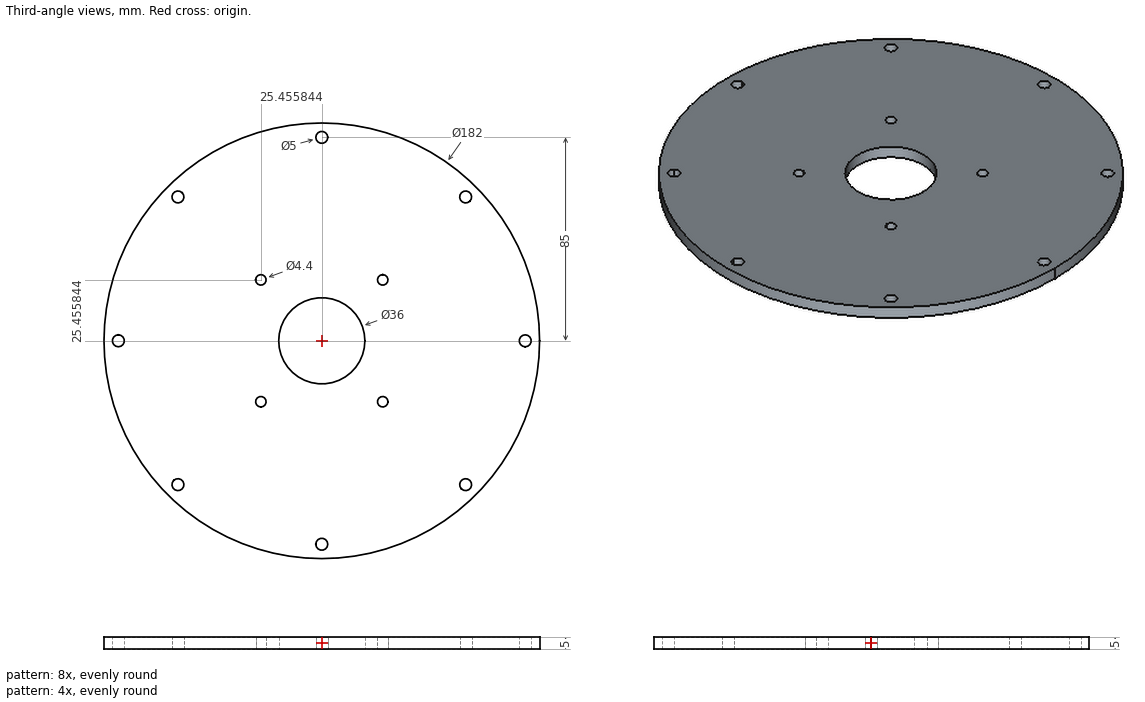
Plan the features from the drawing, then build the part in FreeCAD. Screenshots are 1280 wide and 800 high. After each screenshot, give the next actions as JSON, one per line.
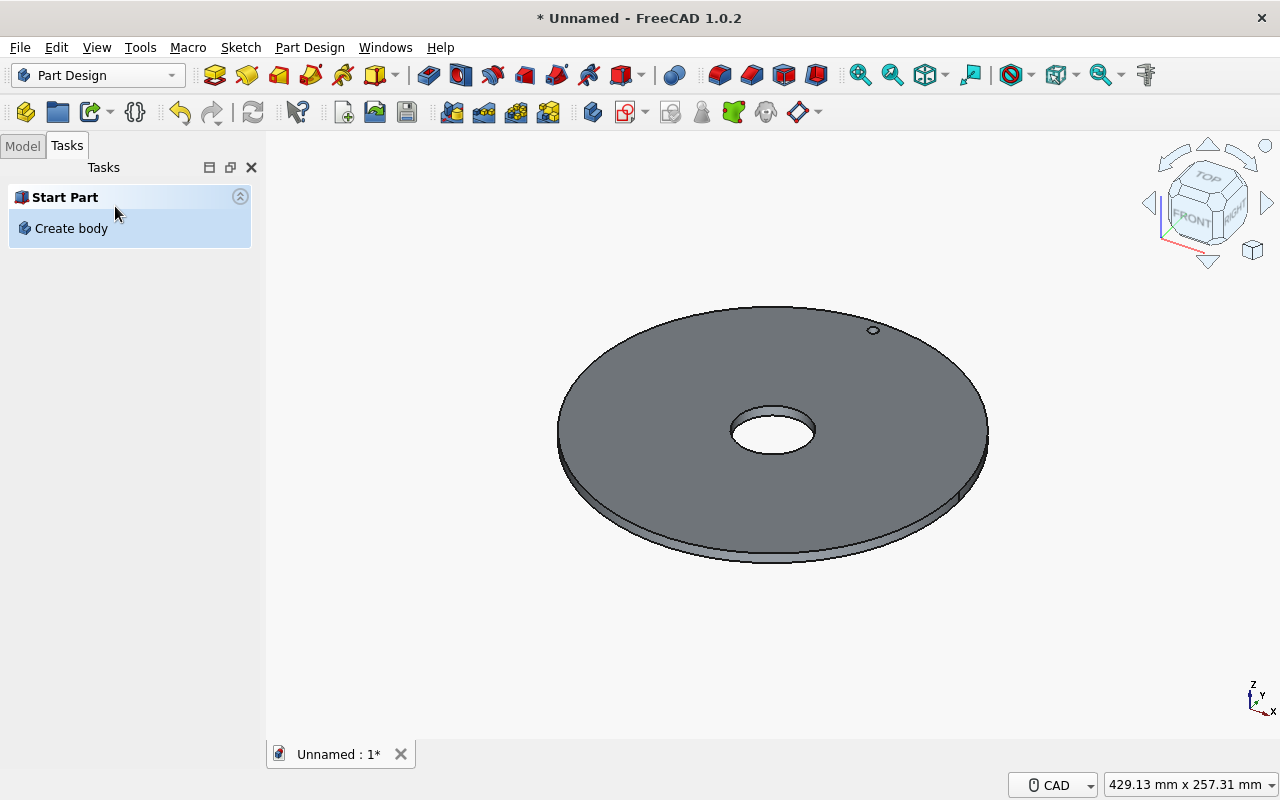
{"action": "left_click", "coordinate": [23, 145]}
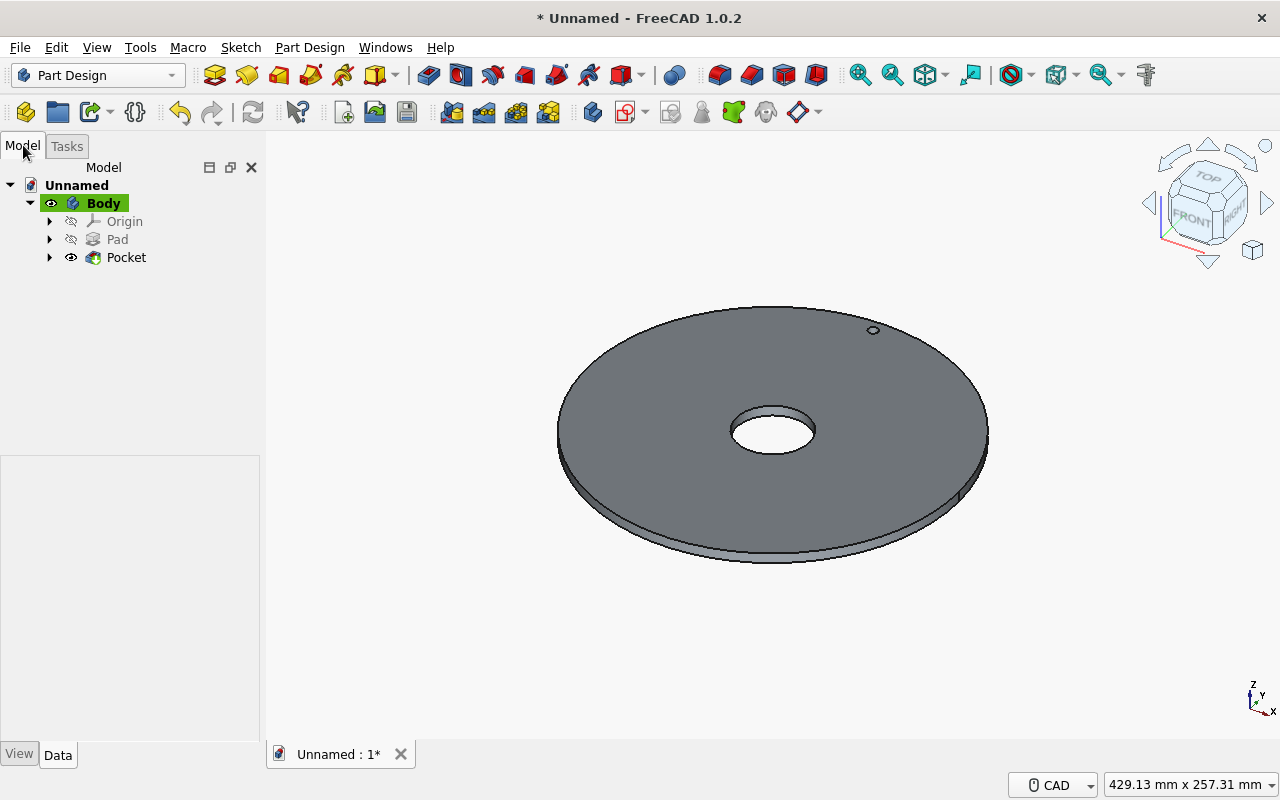
{"action": "left_click", "coordinate": [116, 257]}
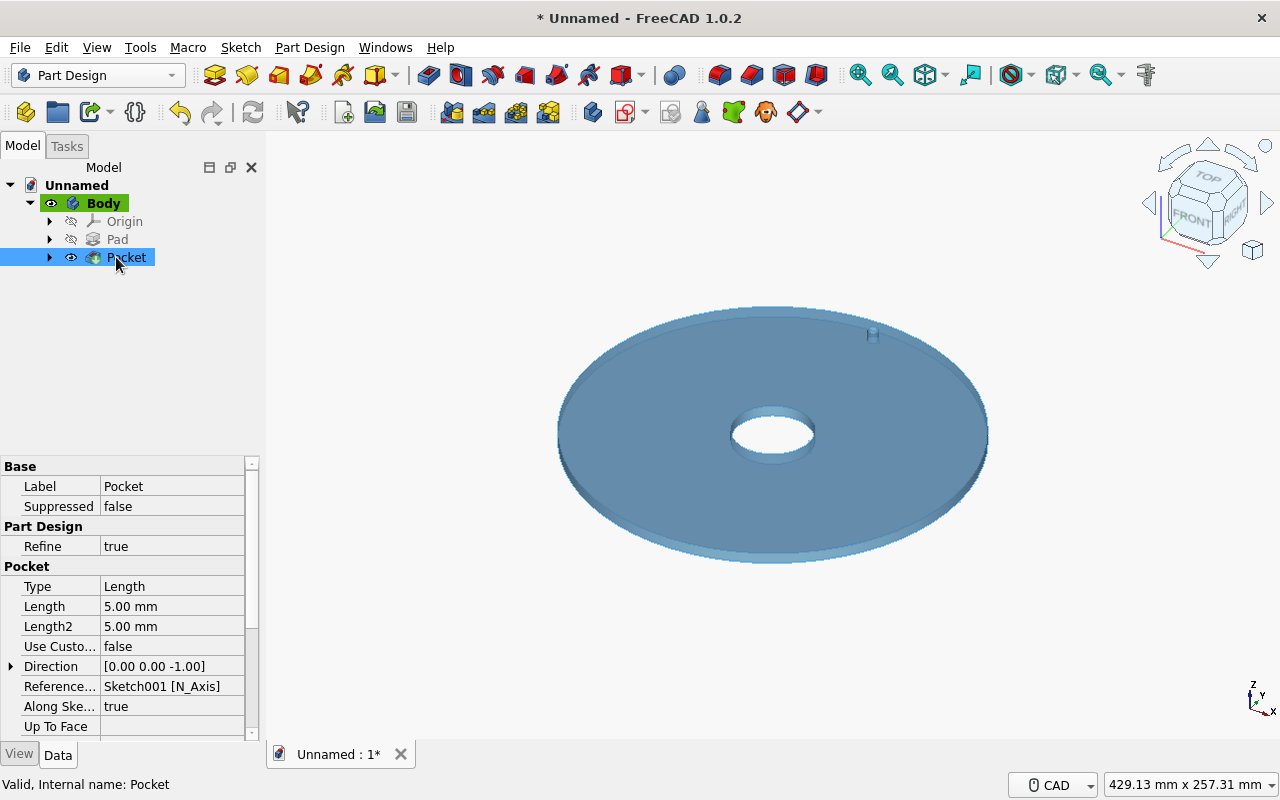
{"action": "left_click", "coordinate": [516, 112]}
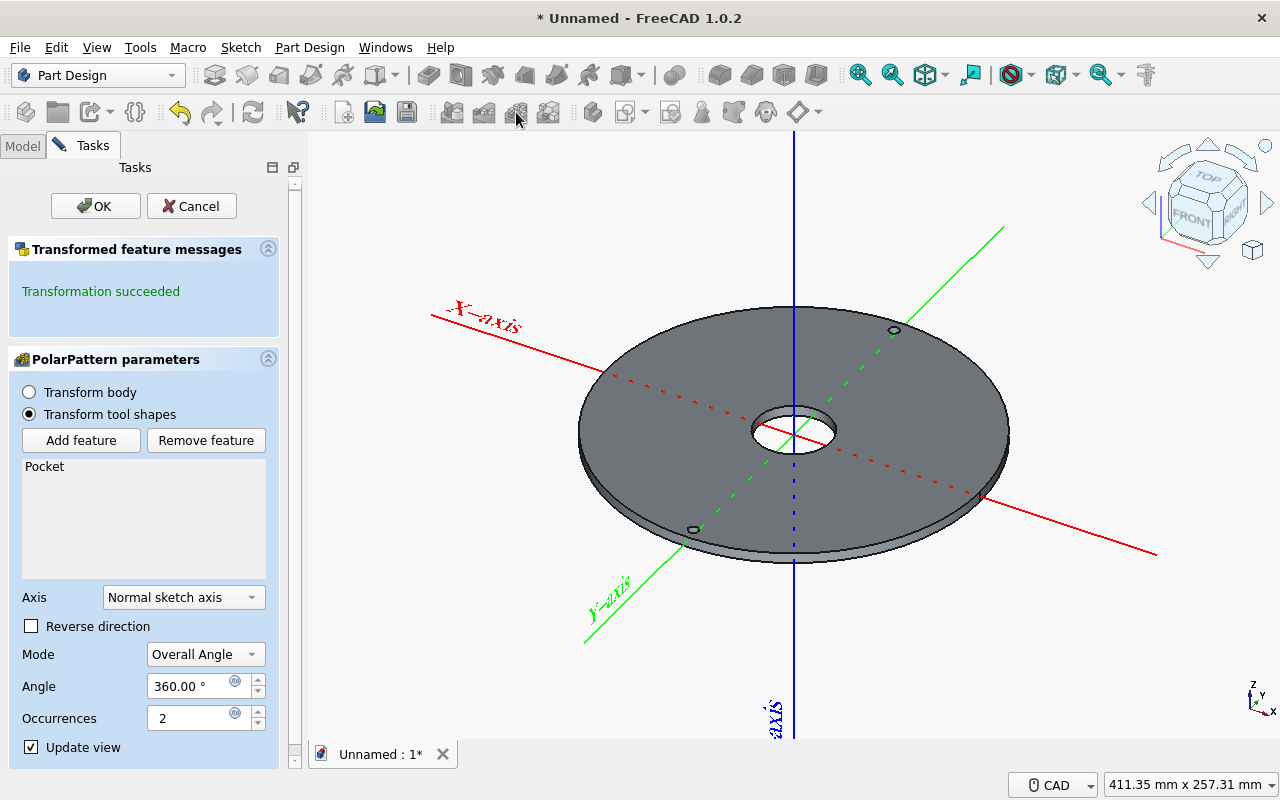
{"action": "left_click", "coordinate": [184, 598]}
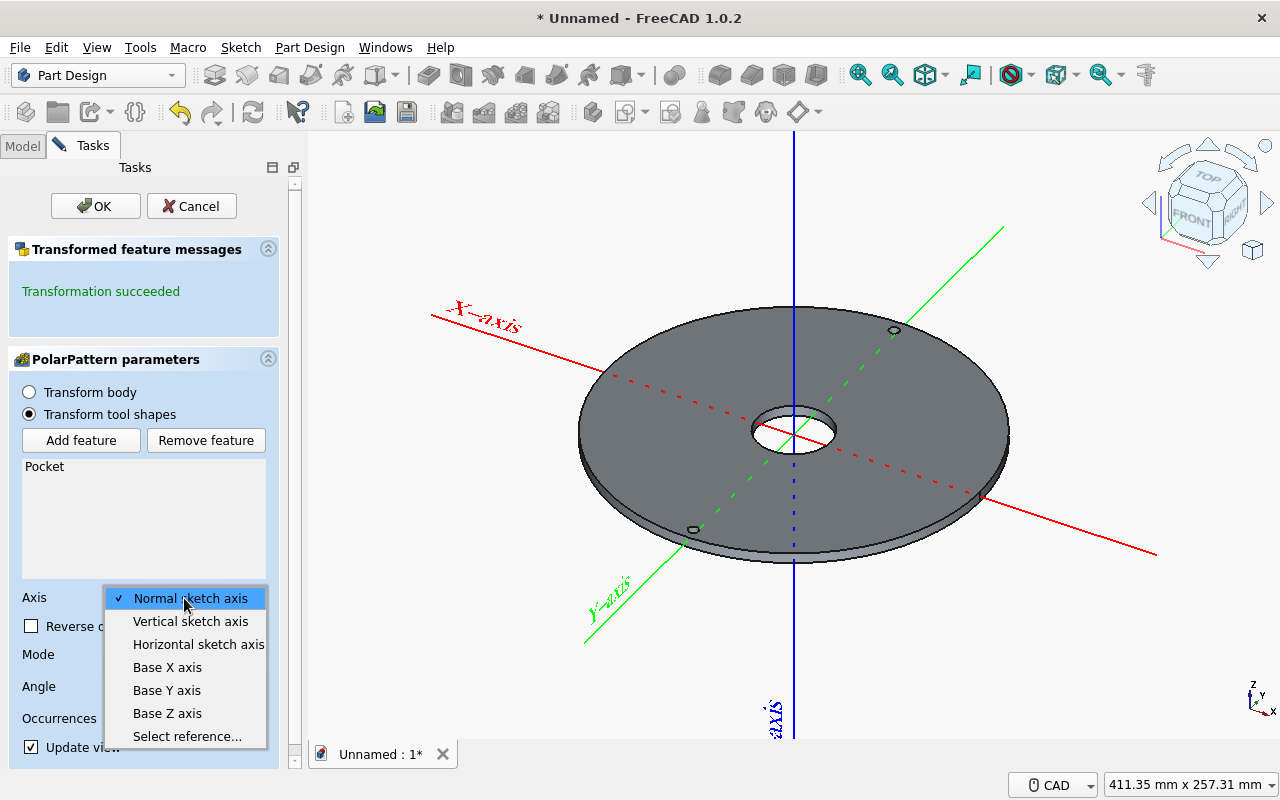
{"action": "left_click", "coordinate": [184, 714]}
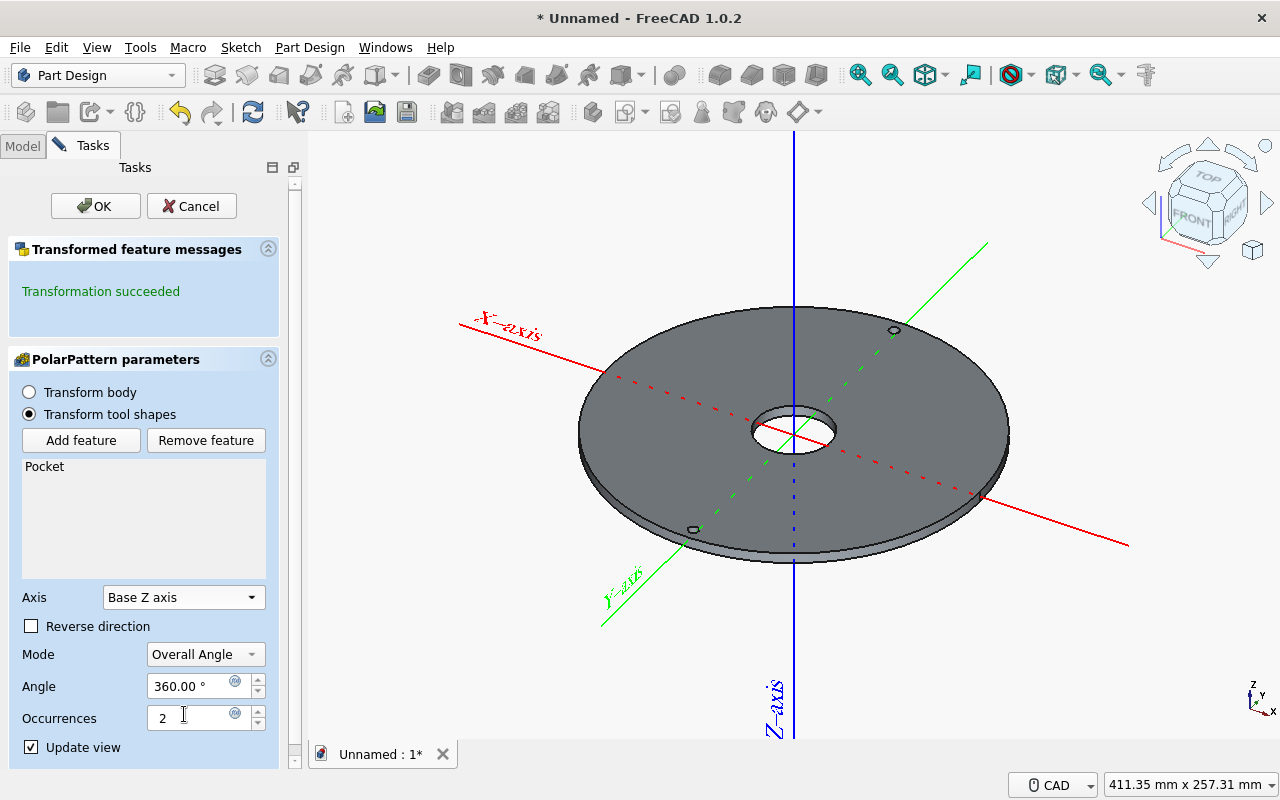
{"action": "triple_click", "coordinate": [198, 718]}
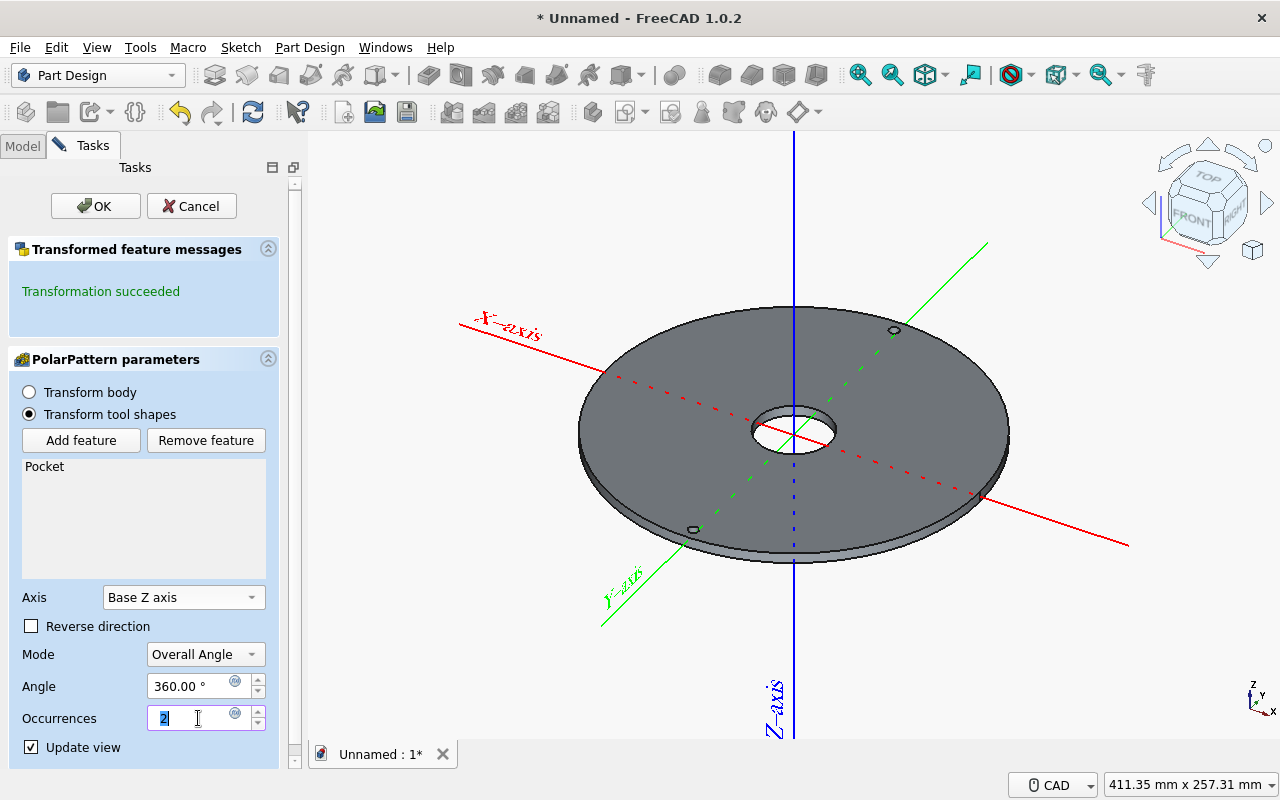
{"action": "type", "text": "8"}
{"action": "key", "text": "Tab"}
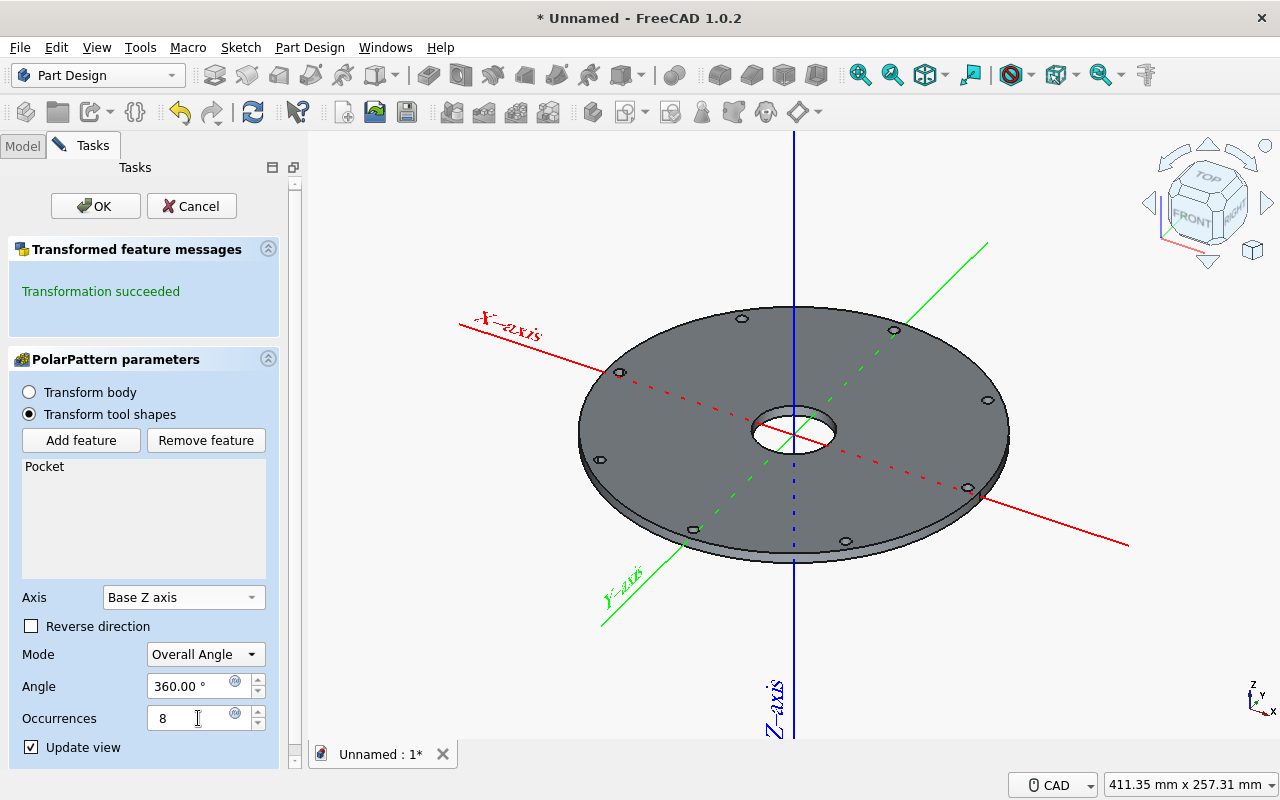
{"action": "left_click", "coordinate": [96, 206]}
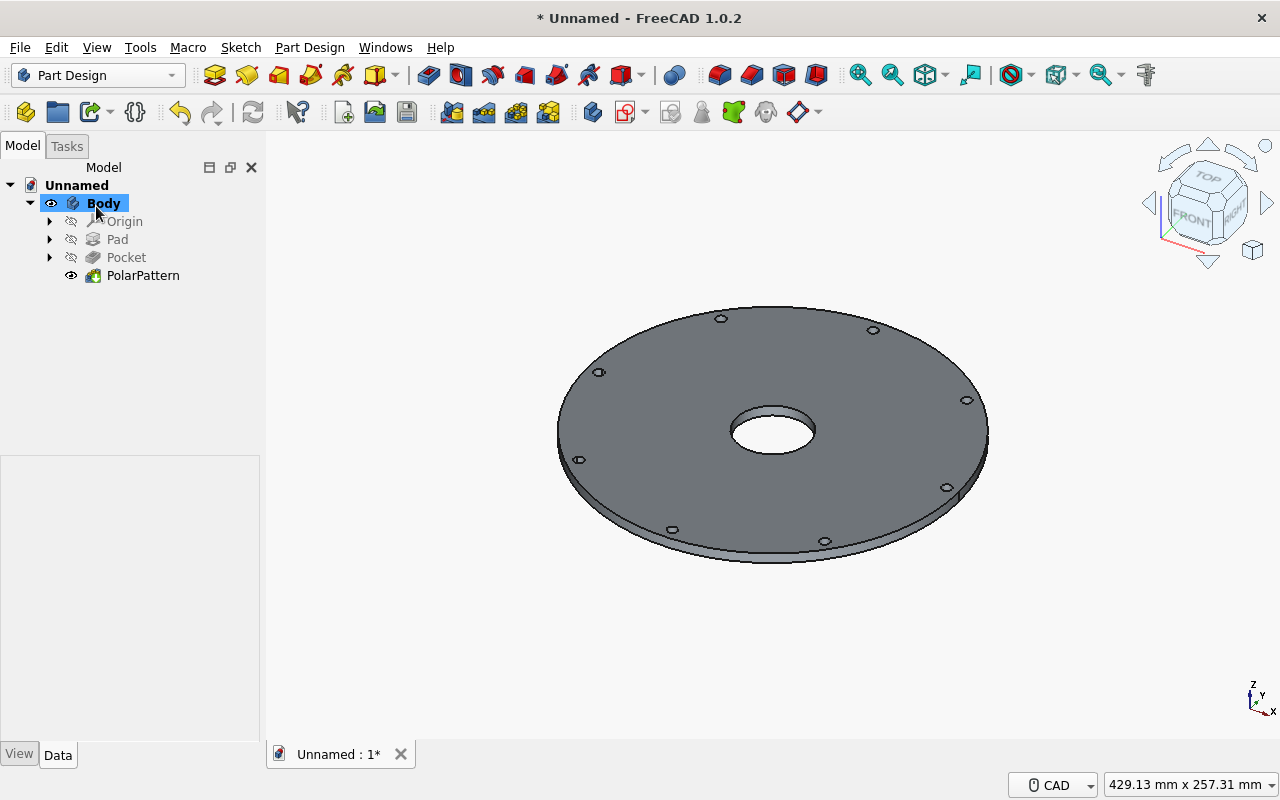
{"action": "key", "text": "5"}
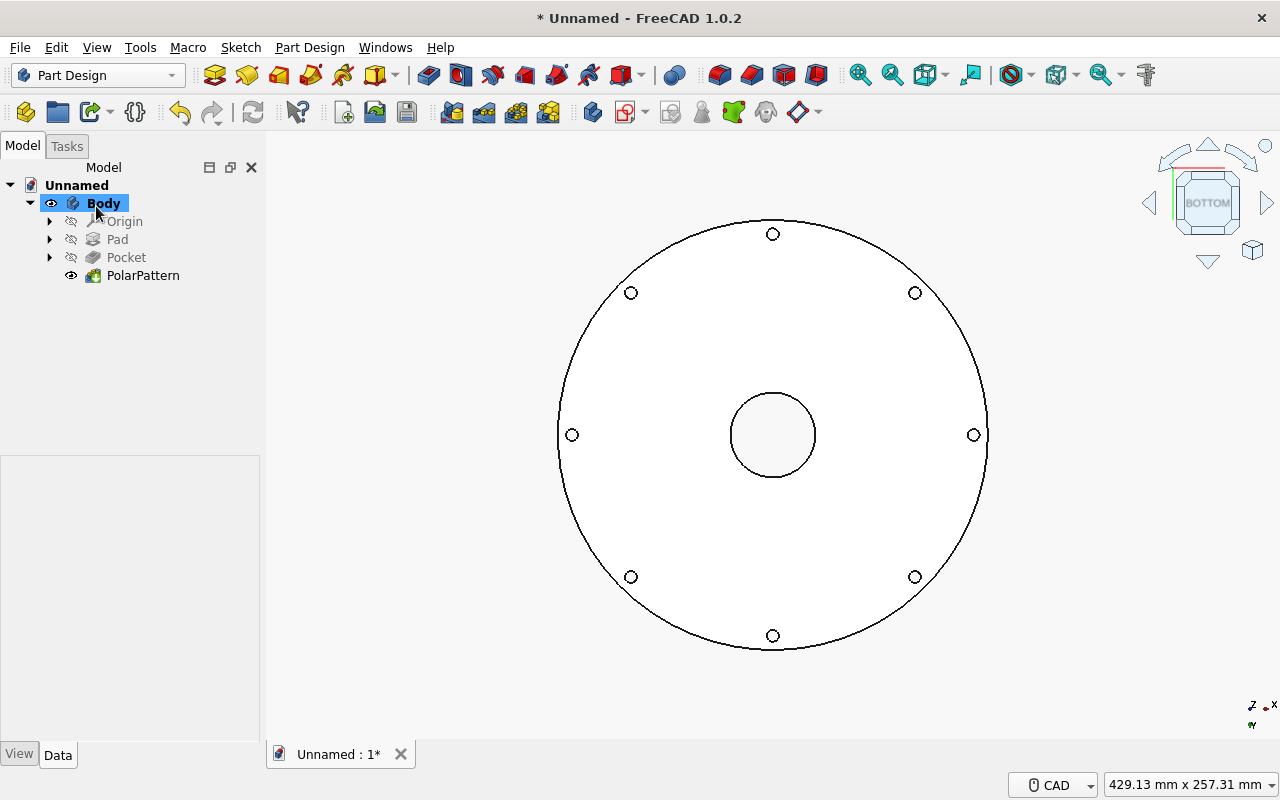
{"action": "left_click", "coordinate": [896, 373]}